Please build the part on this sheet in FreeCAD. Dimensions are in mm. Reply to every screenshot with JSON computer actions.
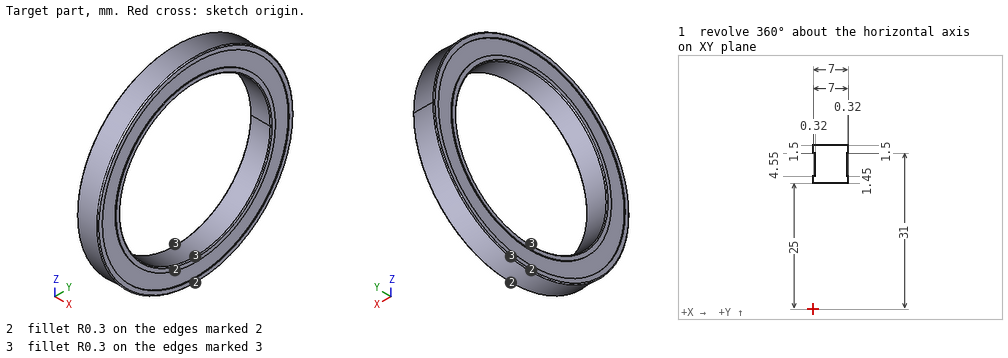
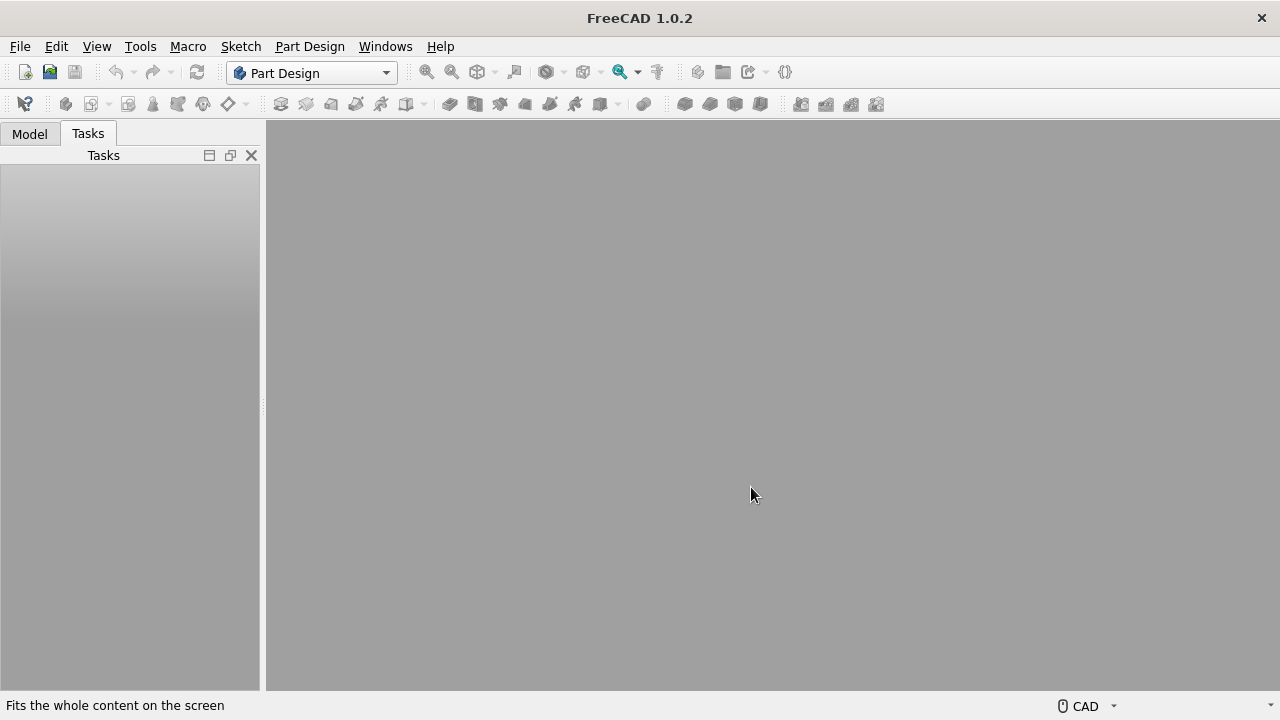
{"action": "key", "text": "ctrl+n"}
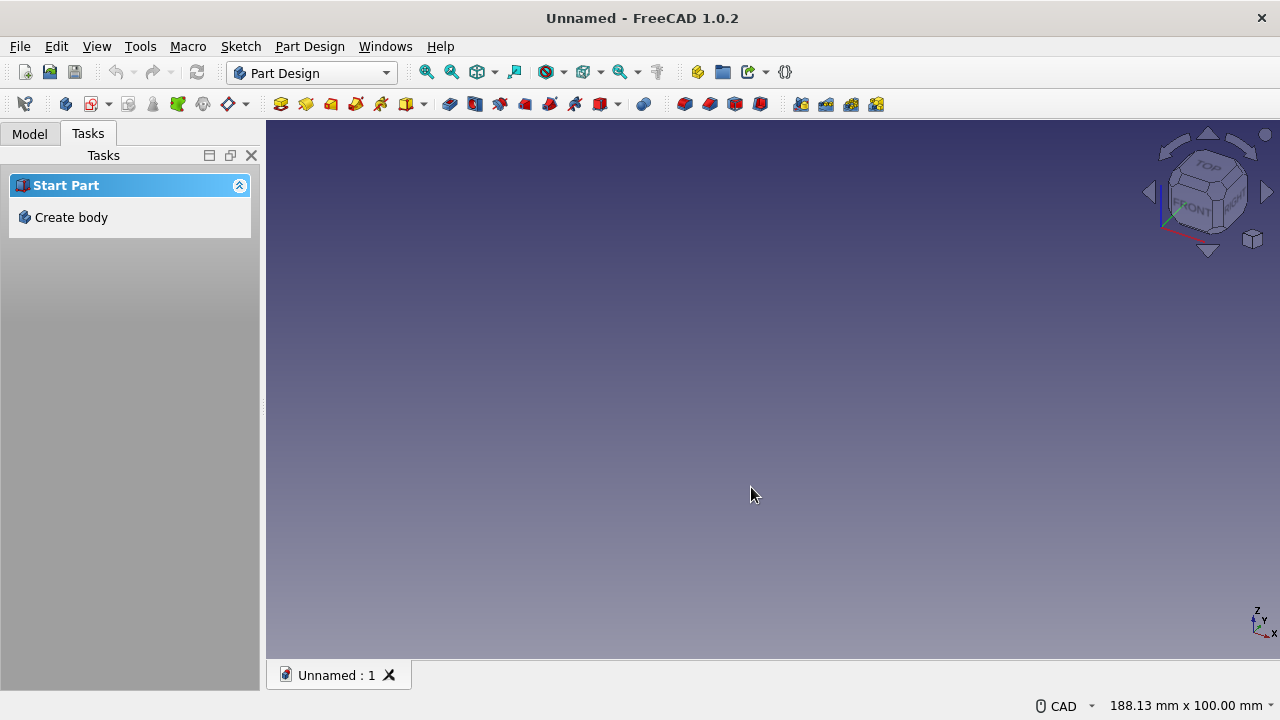
{"action": "left_click", "coordinate": [90, 104]}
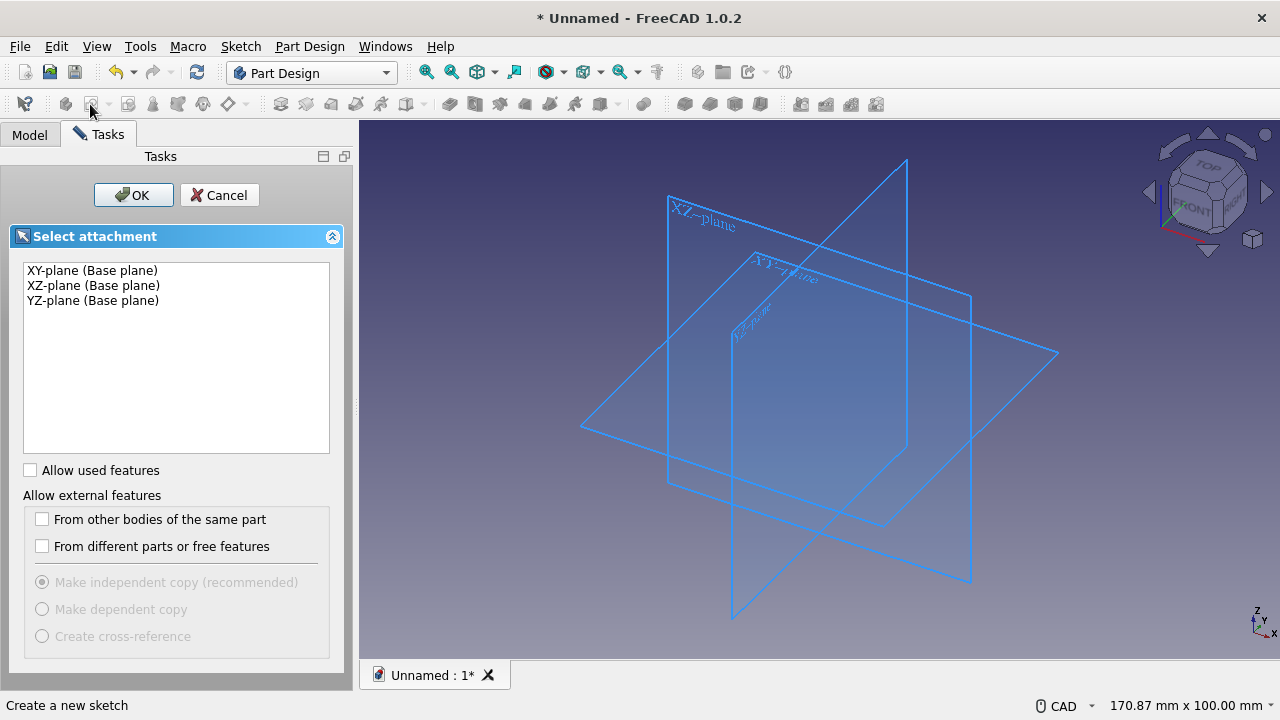
{"action": "left_click", "coordinate": [84, 270]}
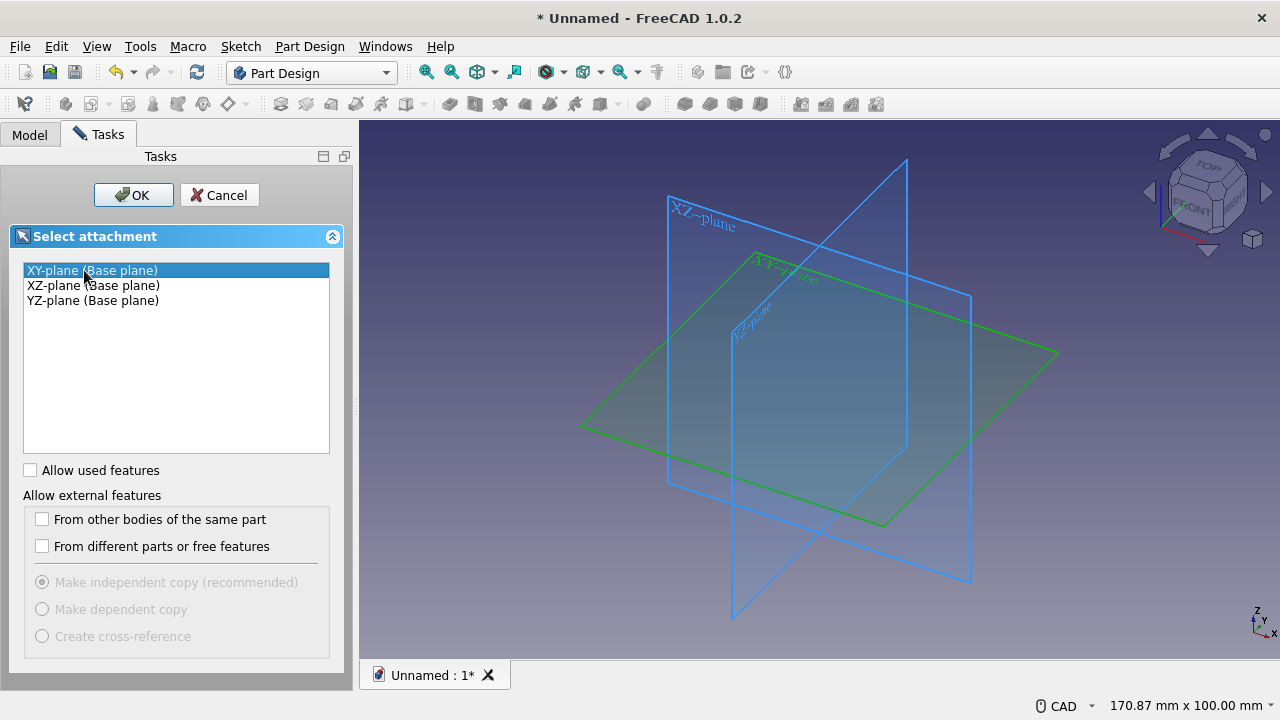
{"action": "left_click", "coordinate": [134, 195]}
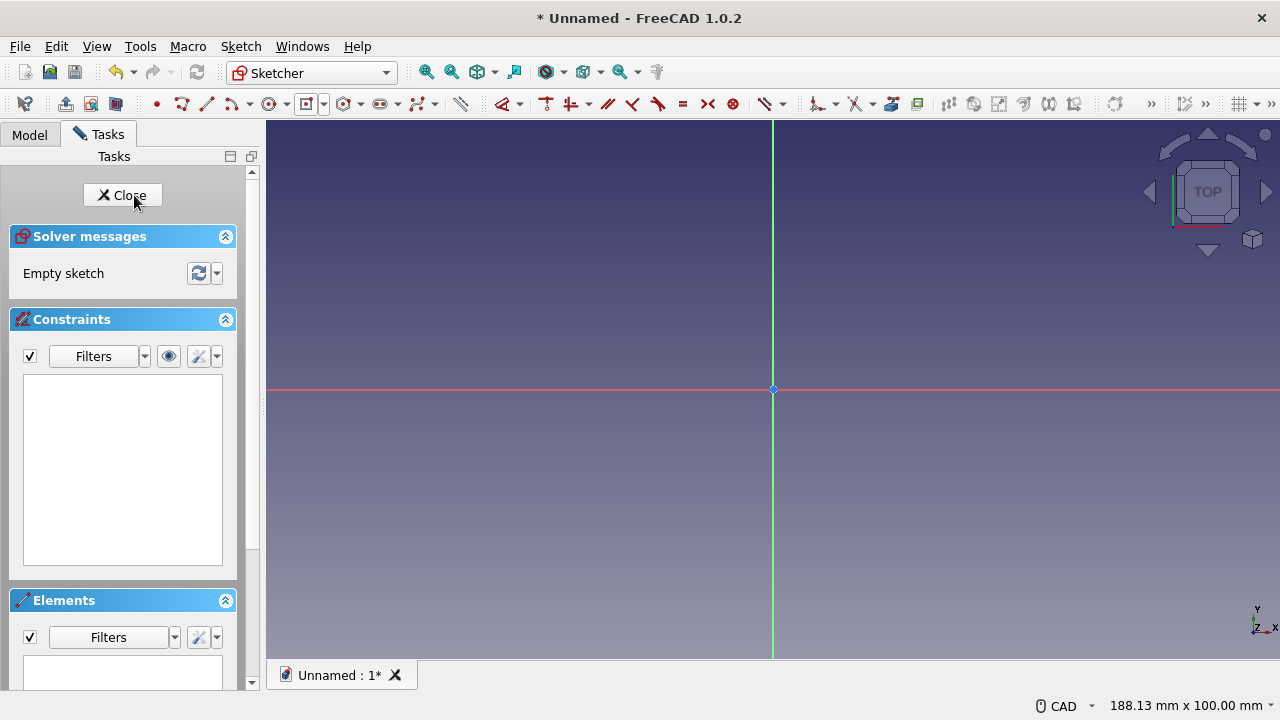
{"action": "scroll", "coordinate": [803, 215], "scroll_direction": "up", "scroll_amount": 11}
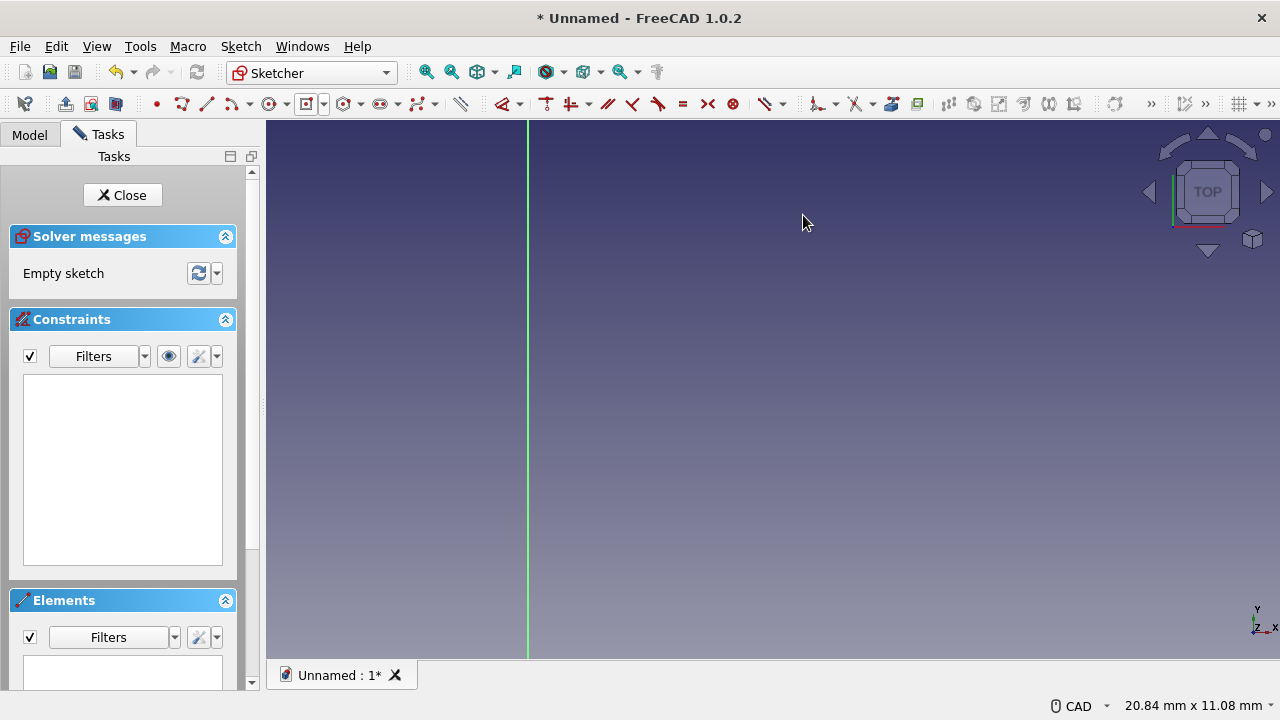
{"action": "left_click", "coordinate": [182, 104]}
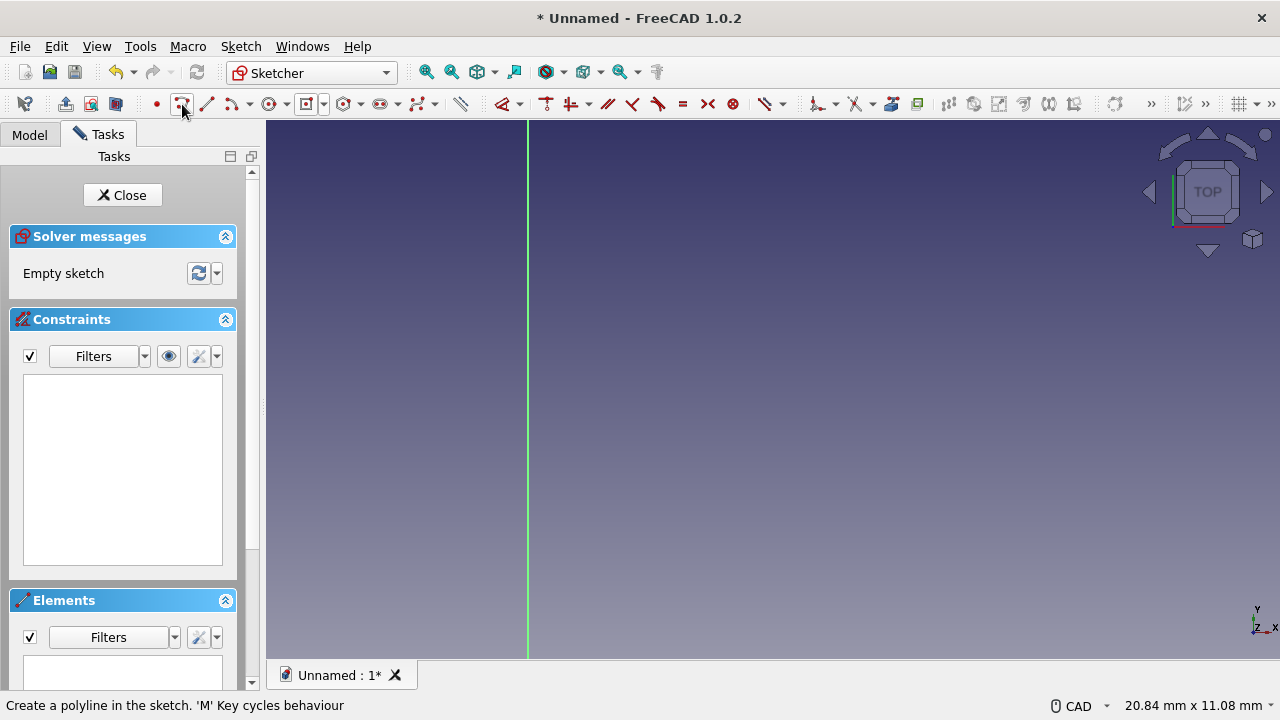
{"action": "left_click", "coordinate": [528, 572]}
{"action": "left_click", "coordinate": [869, 572]}
{"action": "left_click", "coordinate": [869, 502]}
{"action": "left_click", "coordinate": [853, 502]}
{"action": "left_click", "coordinate": [853, 280]}
{"action": "left_click", "coordinate": [869, 280]}
{"action": "left_click", "coordinate": [869, 207]}
{"action": "left_click", "coordinate": [528, 207]}
{"action": "left_click", "coordinate": [537, 280]}
{"action": "left_click", "coordinate": [544, 280]}
{"action": "left_click", "coordinate": [544, 502]}
{"action": "left_click", "coordinate": [537, 502]}
{"action": "left_click", "coordinate": [528, 573]}
{"action": "key", "text": "Escape"}
{"action": "key", "text": "Escape"}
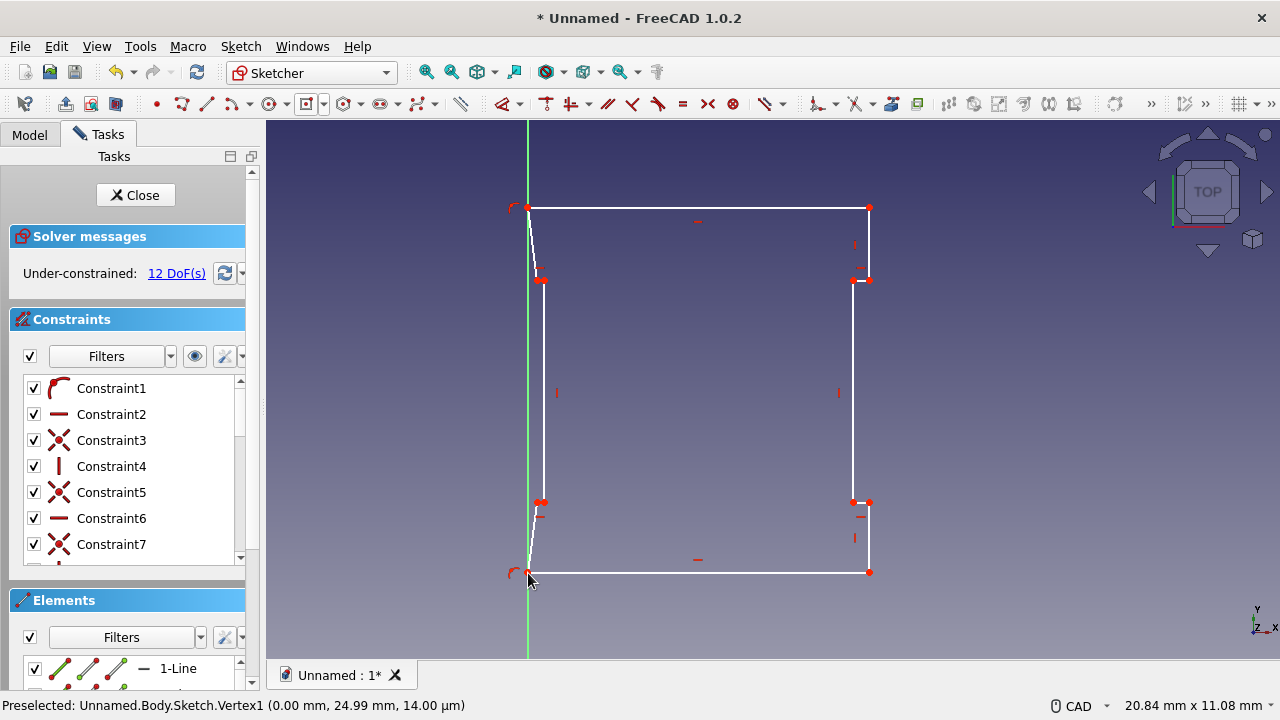
{"action": "left_click", "coordinate": [531, 230]}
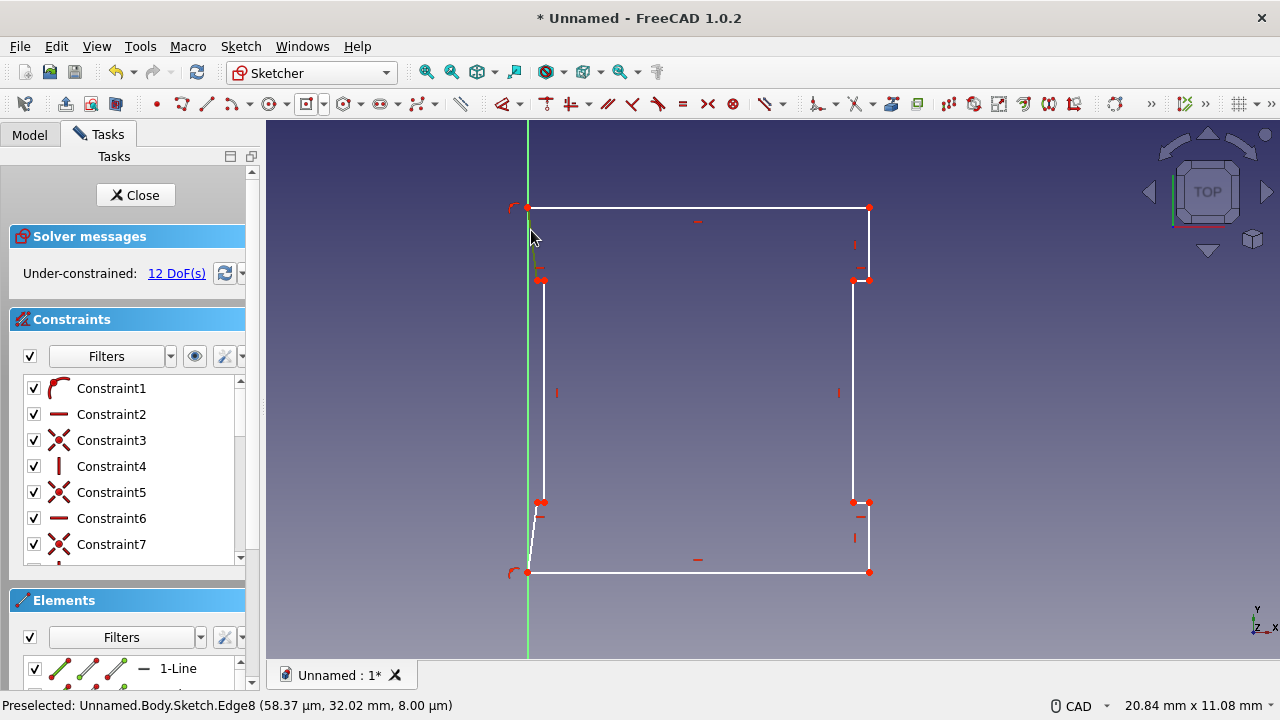
{"action": "left_click", "coordinate": [588, 104]}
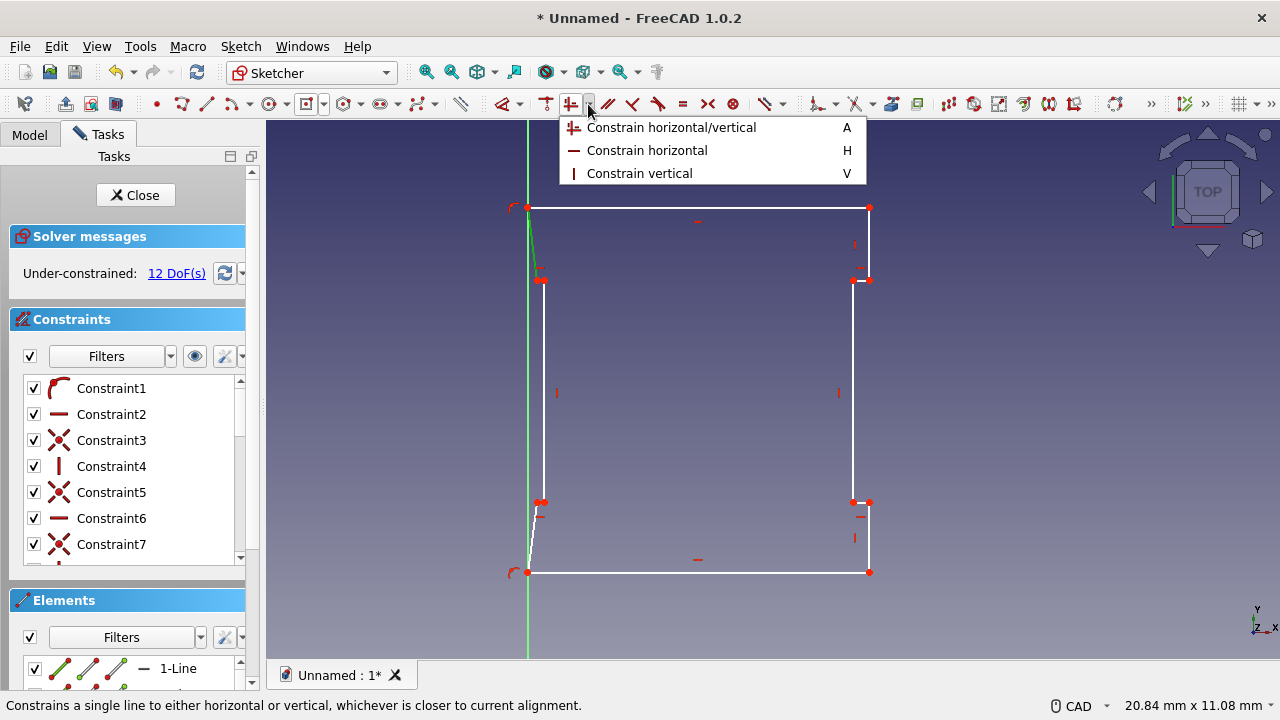
{"action": "left_click", "coordinate": [713, 174]}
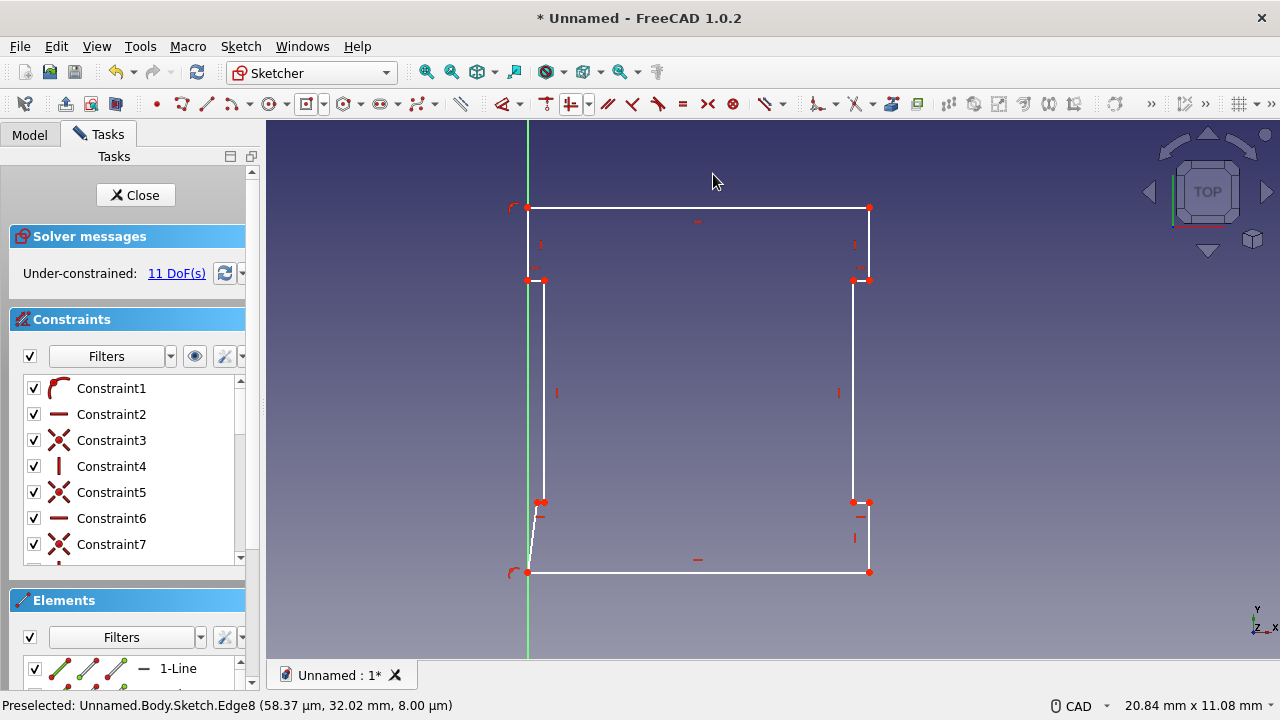
{"action": "left_click", "coordinate": [531, 552]}